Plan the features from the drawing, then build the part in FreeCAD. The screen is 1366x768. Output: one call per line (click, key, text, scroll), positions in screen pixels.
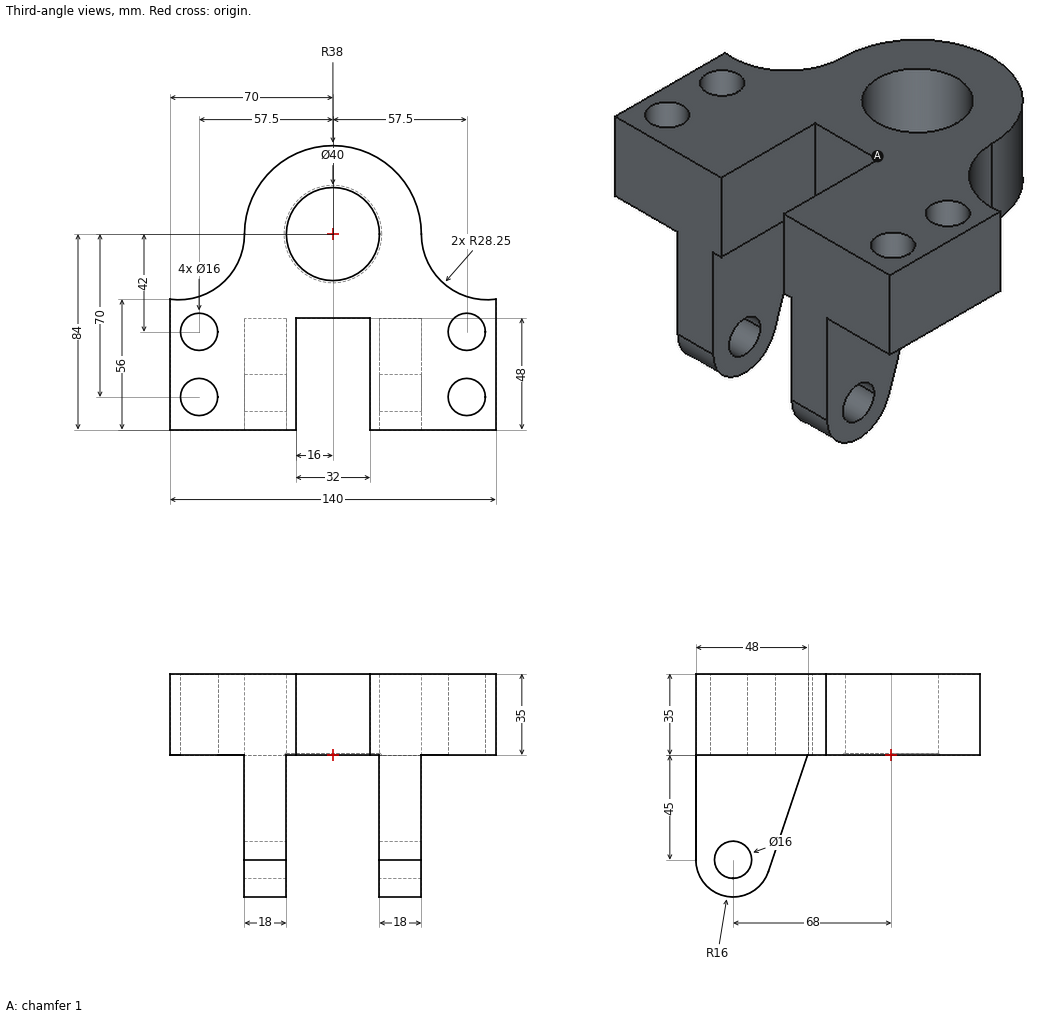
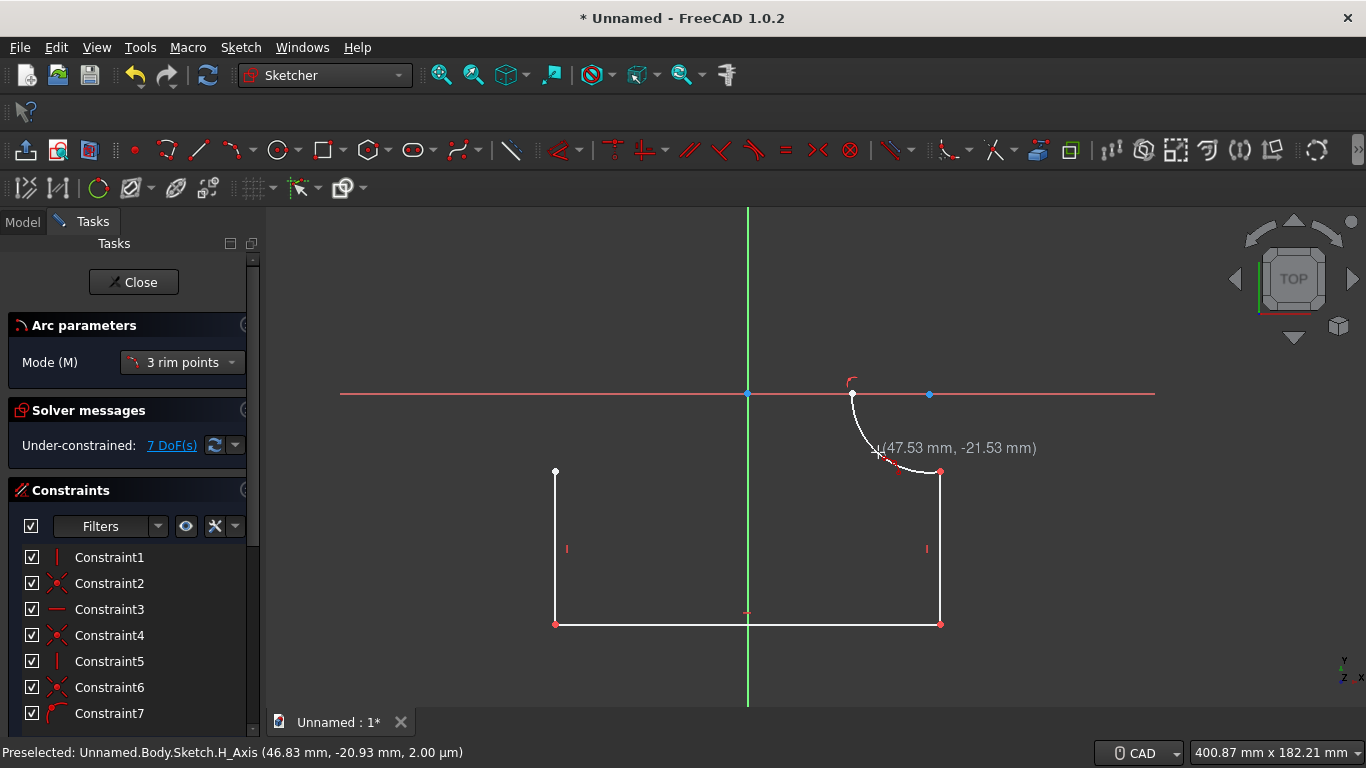
click(852, 394)
click(643, 394)
click(780, 295)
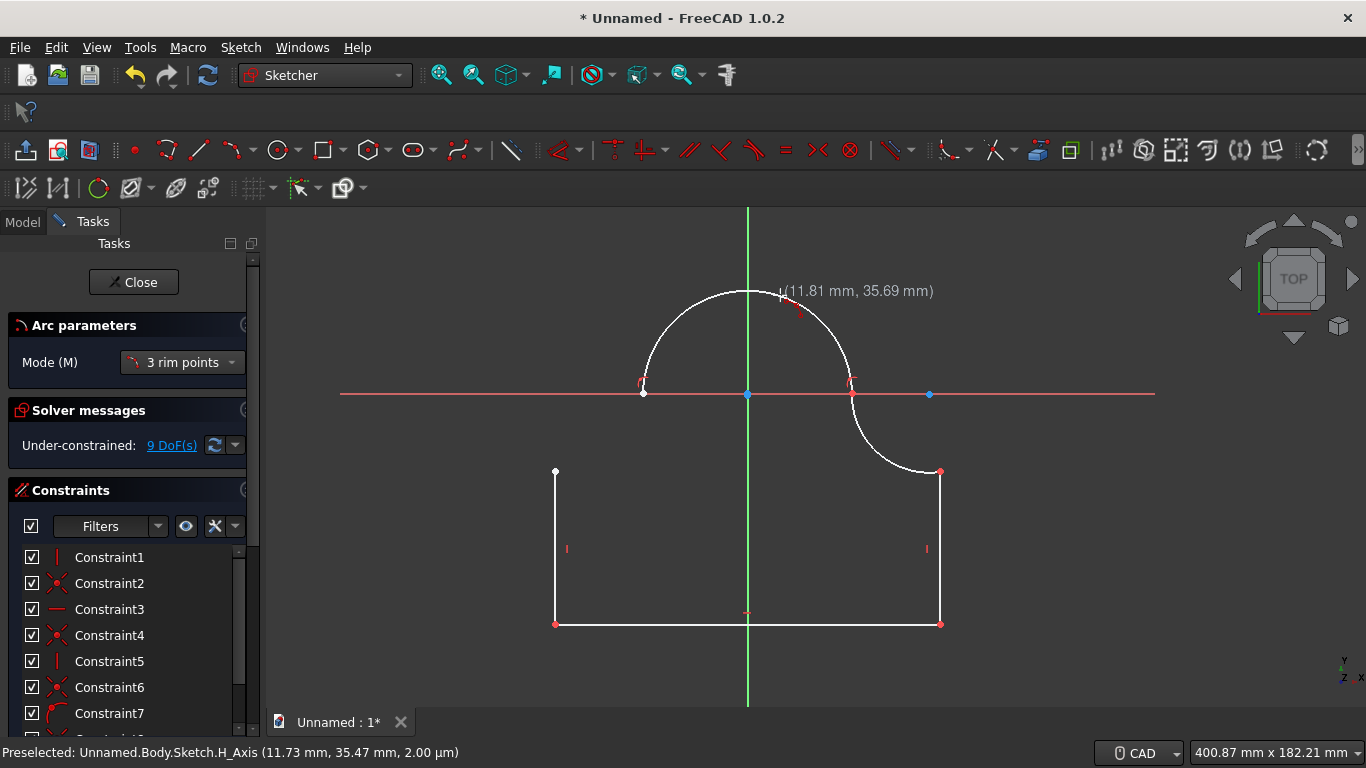
click(643, 394)
click(555, 472)
click(617, 452)
key(Escape)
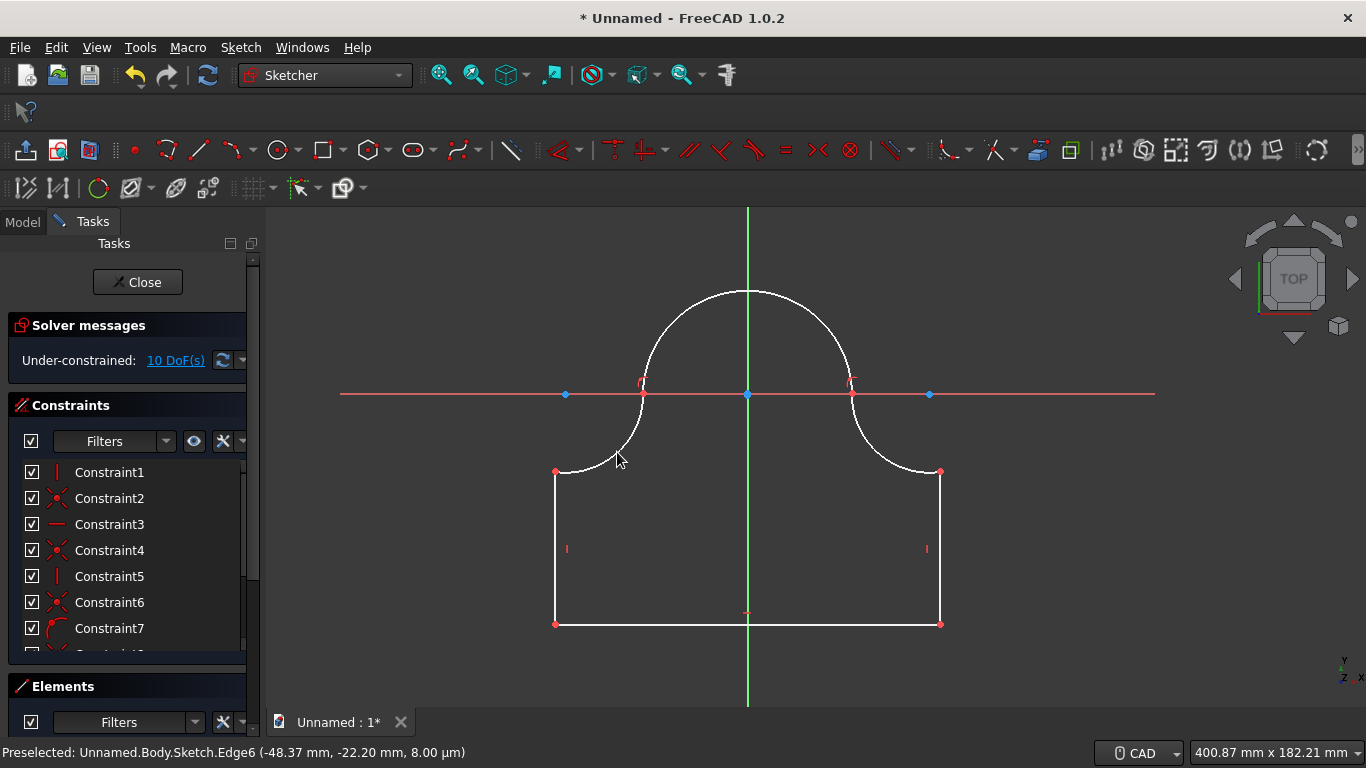
click(862, 432)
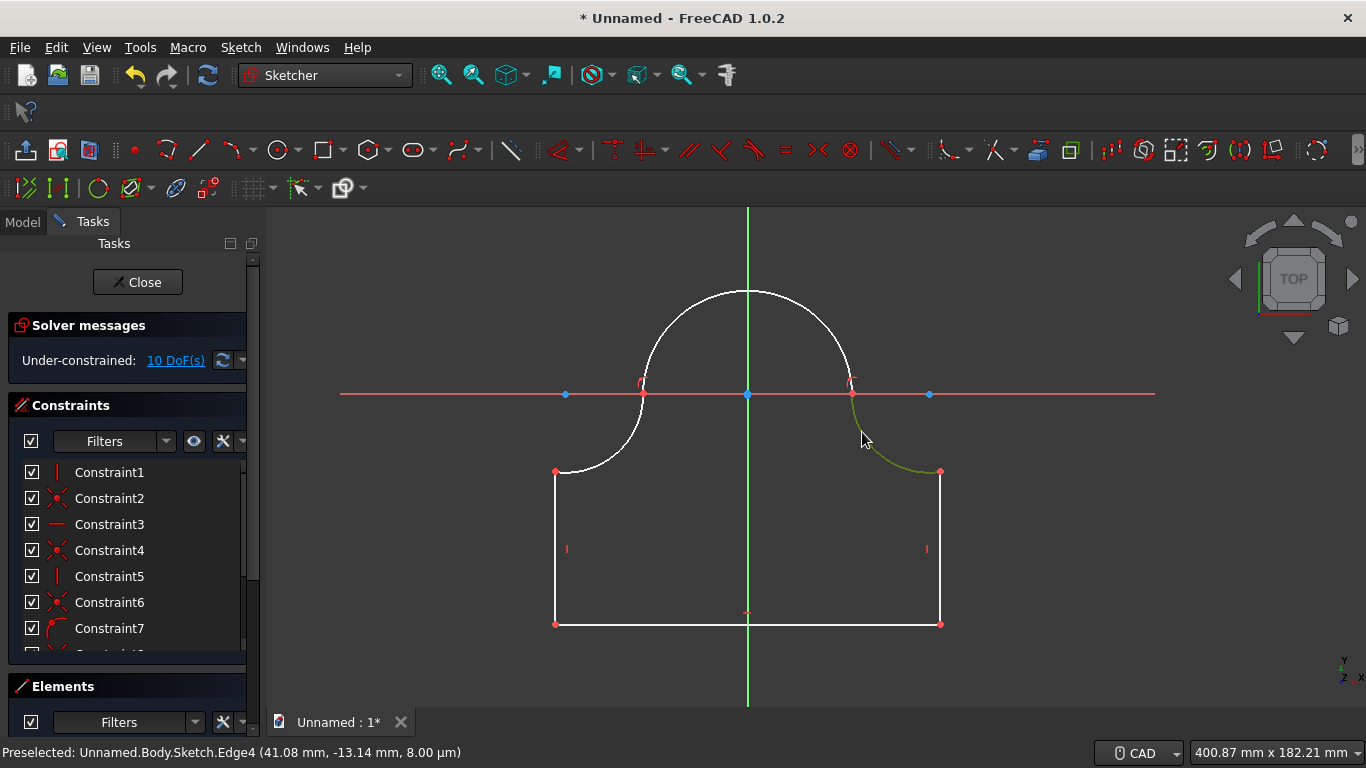
click(808, 310)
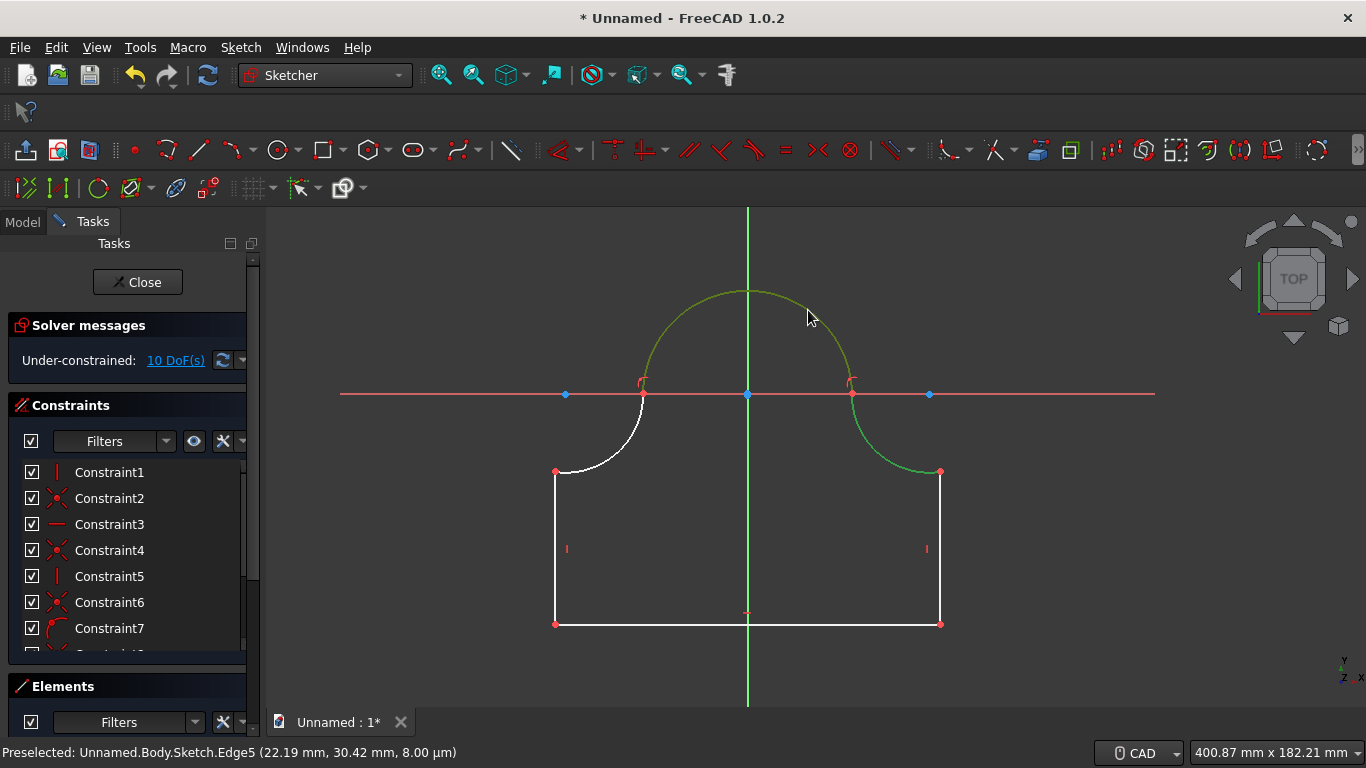
key(t)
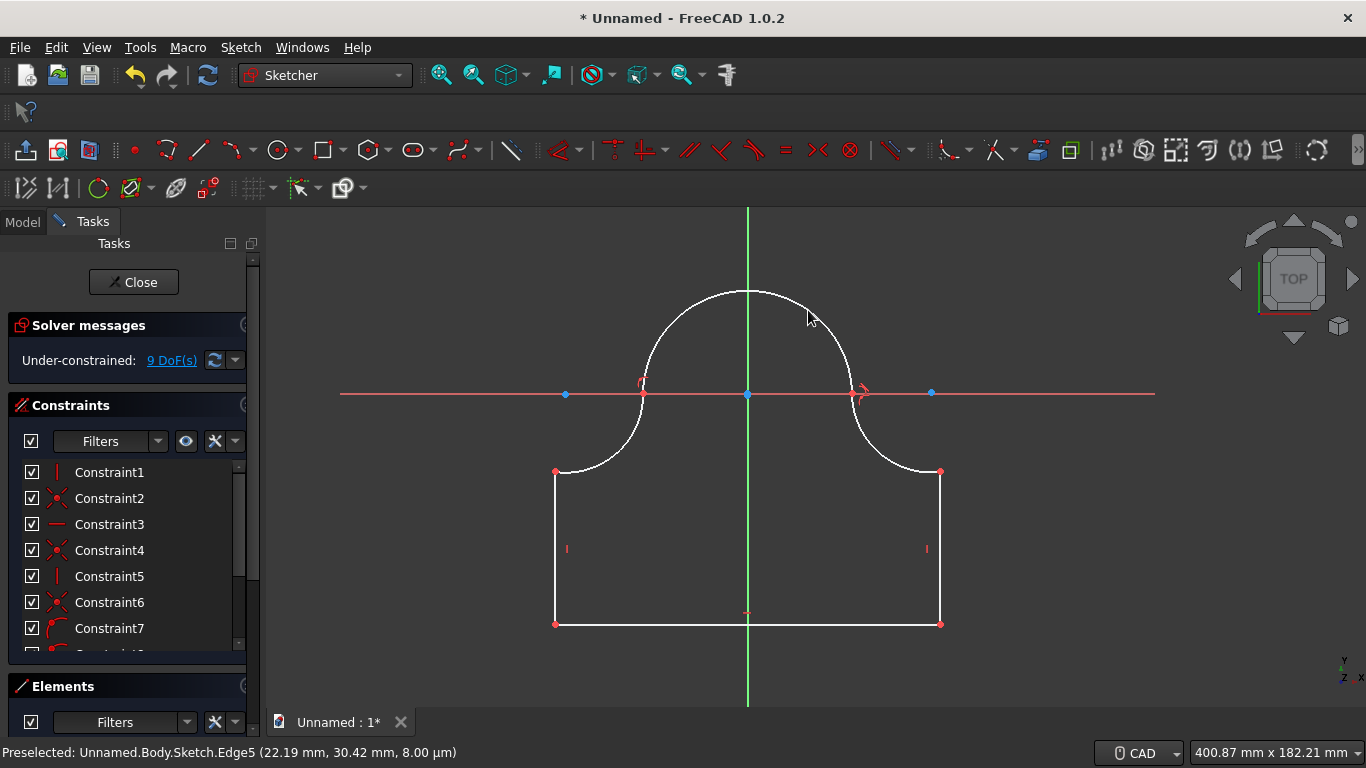
click(808, 310)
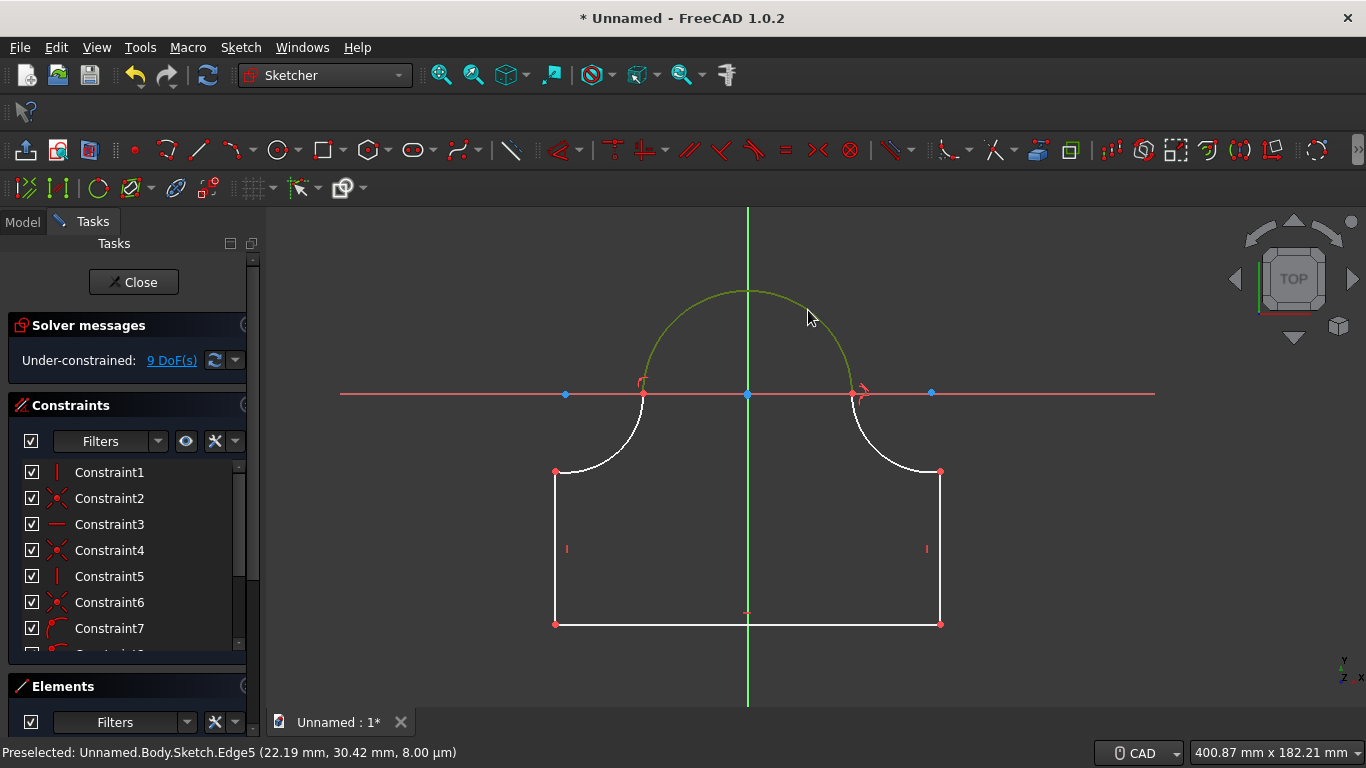
click(594, 467)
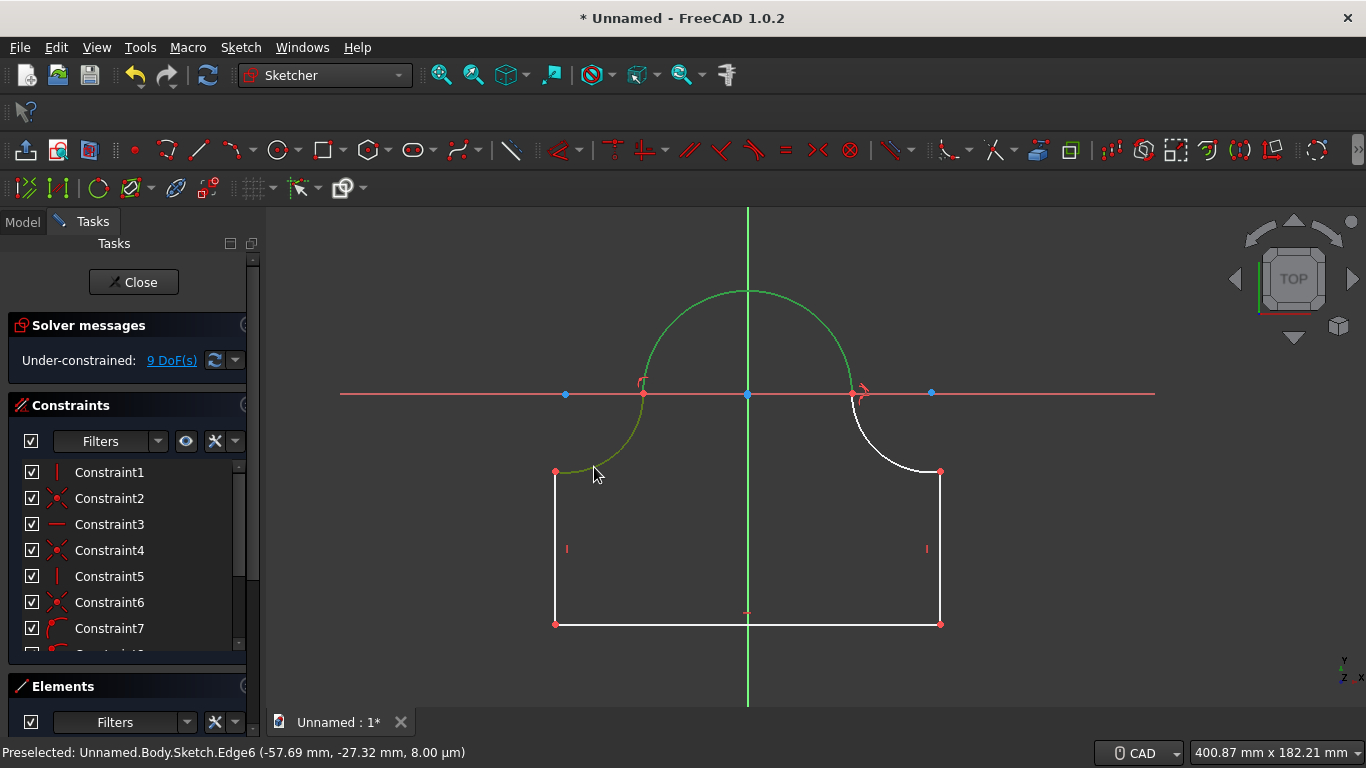
key(t)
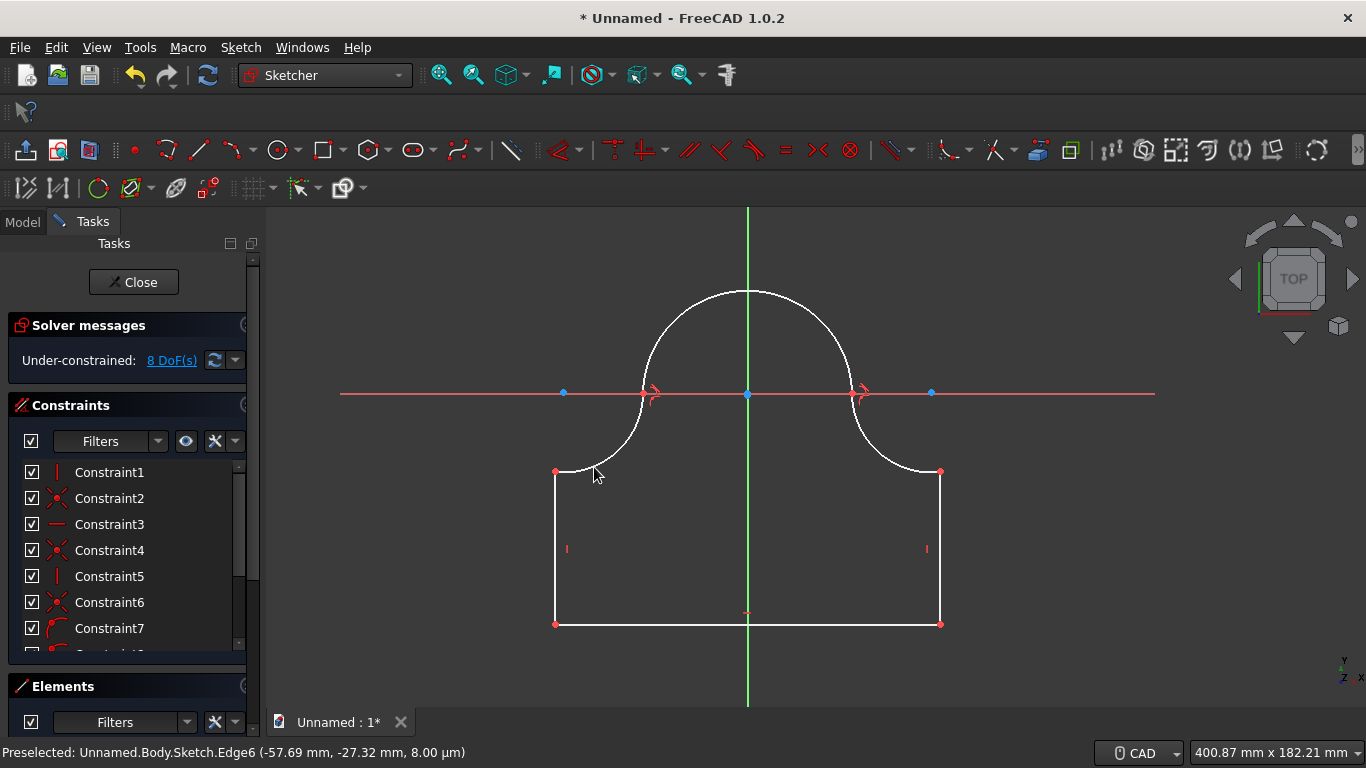
drag(738, 384, 758, 405)